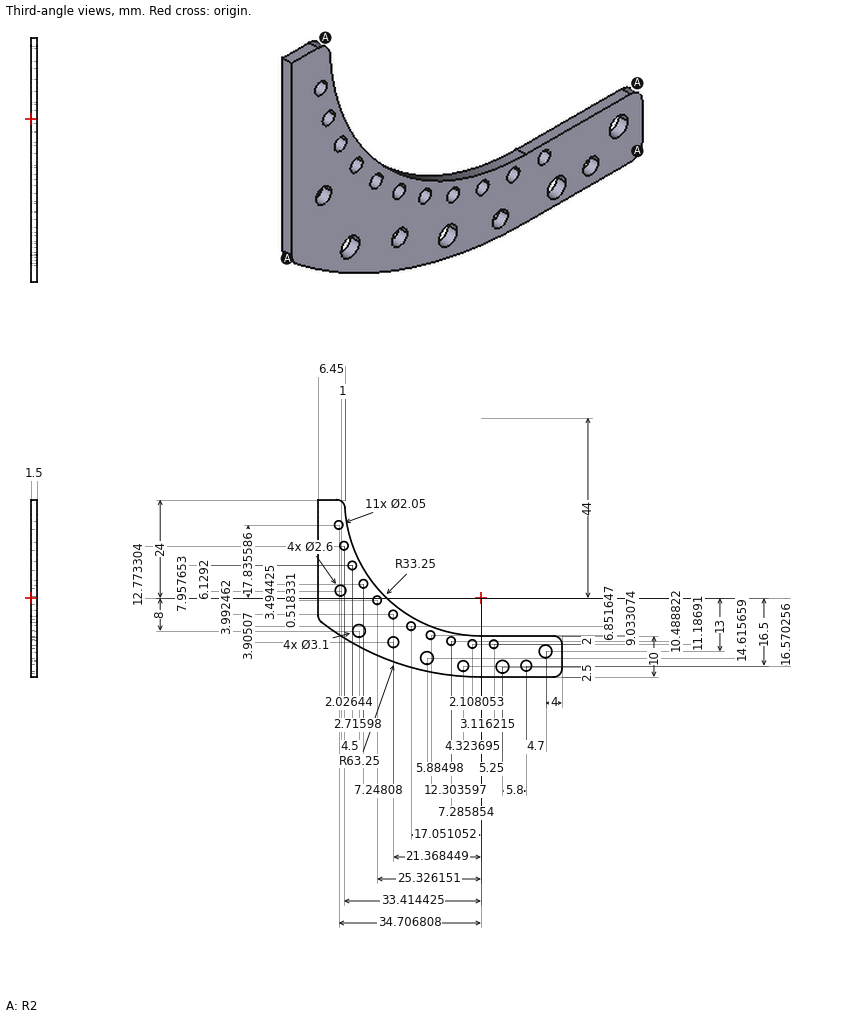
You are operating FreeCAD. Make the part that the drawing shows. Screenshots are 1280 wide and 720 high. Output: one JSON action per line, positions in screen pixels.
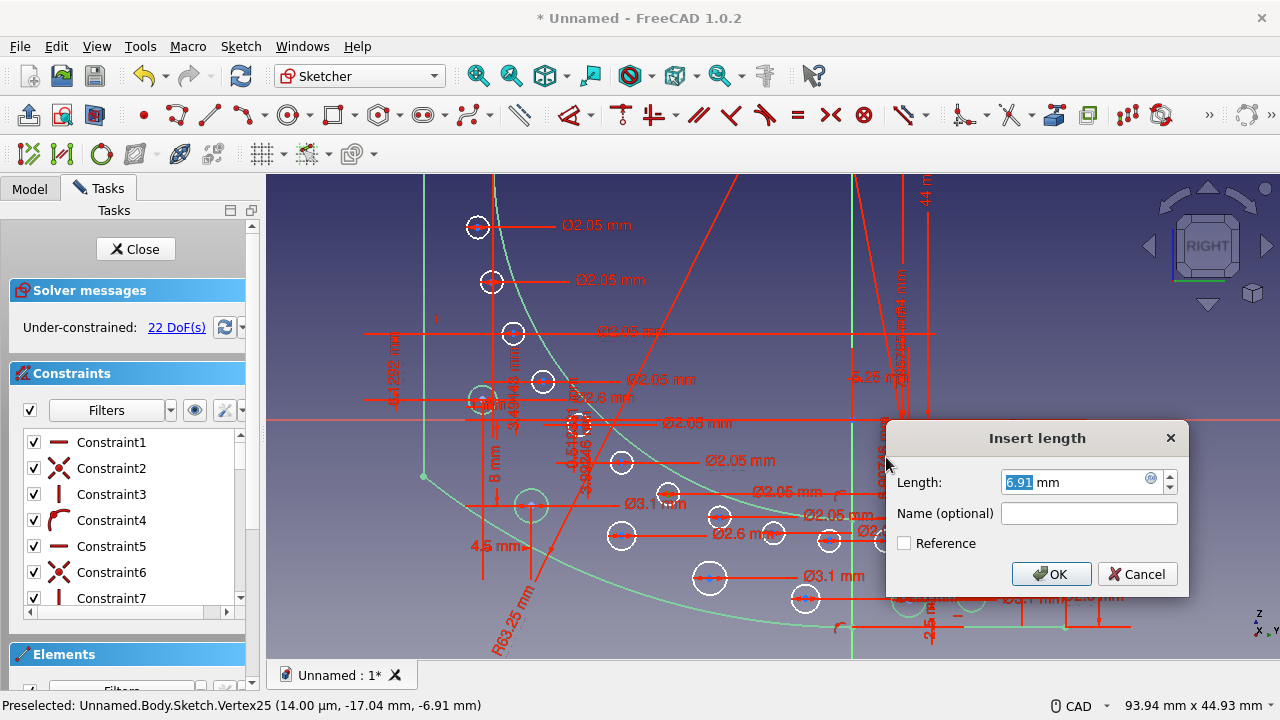
{"action": "type", "text": "6.851647"}
{"action": "key", "text": "Return"}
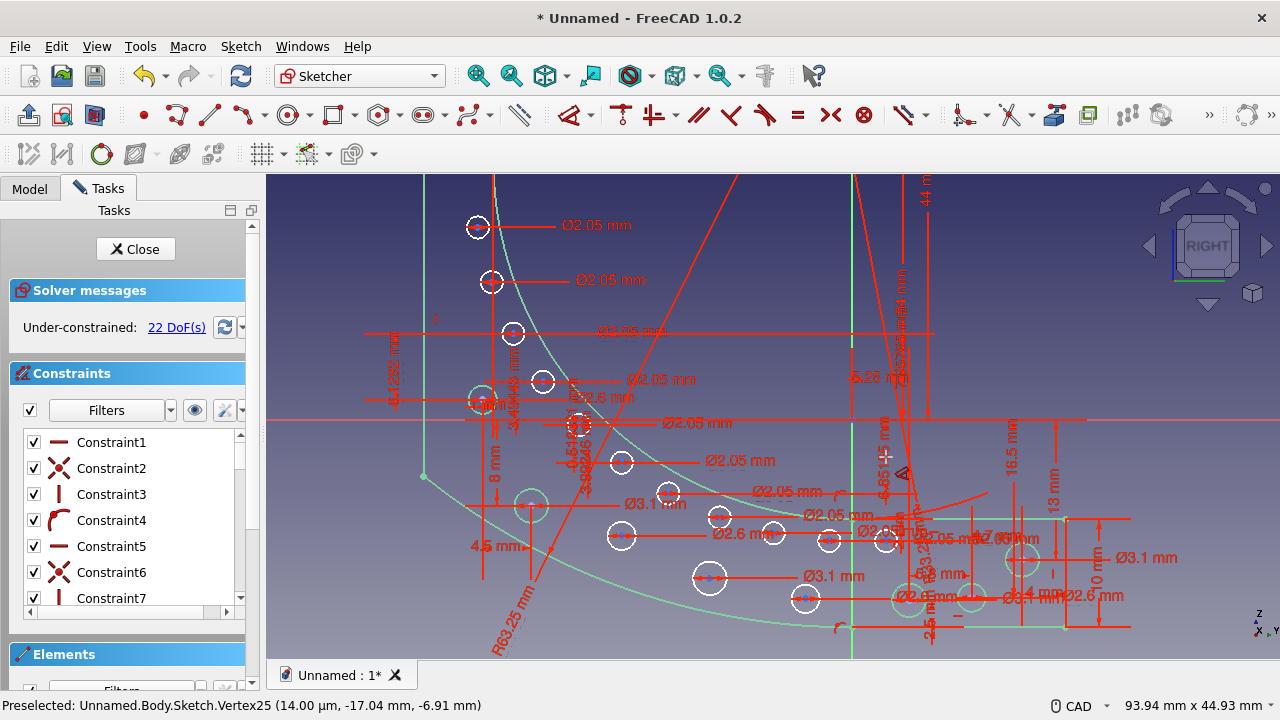
{"action": "left_click", "coordinate": [720, 517]}
{"action": "left_click", "coordinate": [886, 491]}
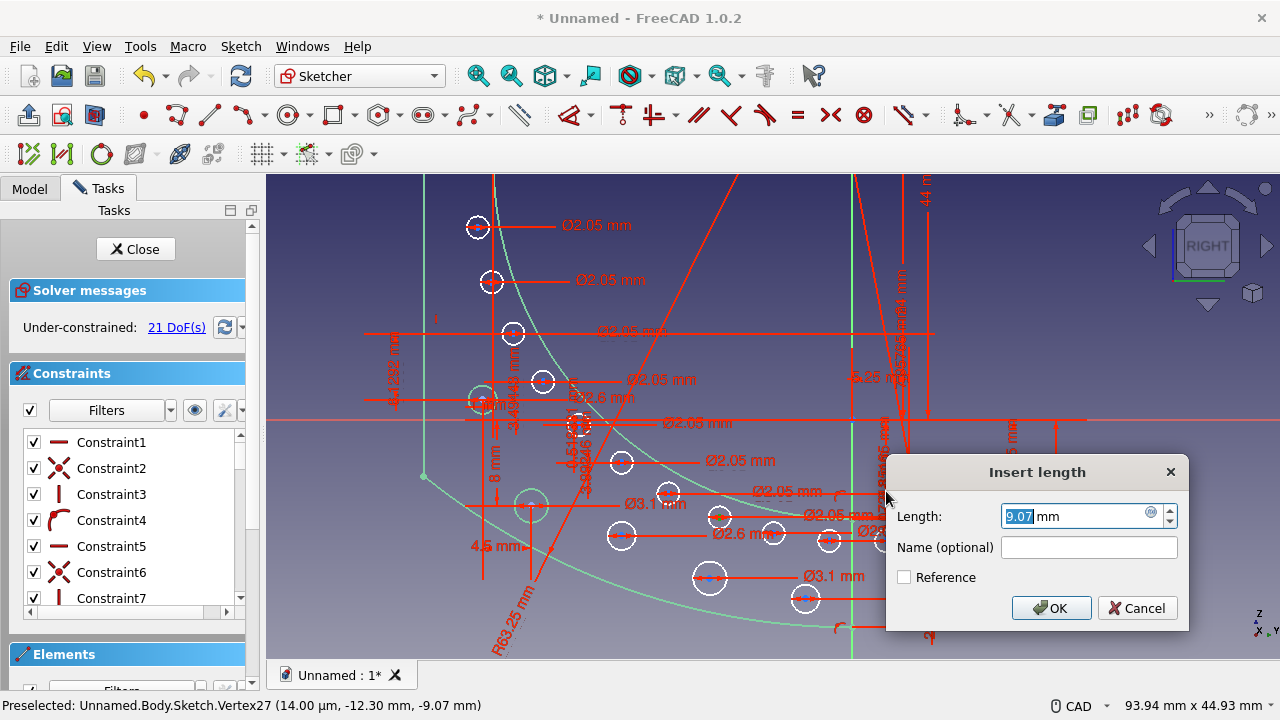
{"action": "type", "text": "9.033074"}
{"action": "key", "text": "Return"}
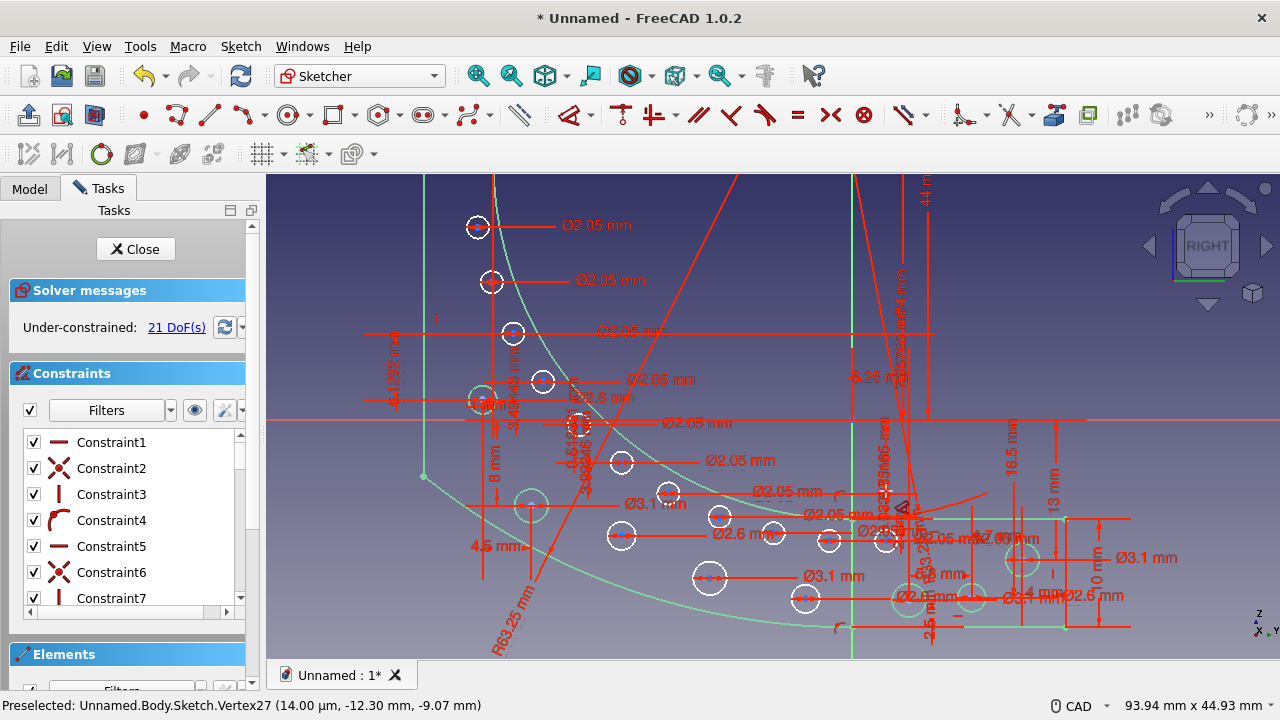
{"action": "left_click", "coordinate": [774, 533]}
{"action": "left_click", "coordinate": [813, 567]}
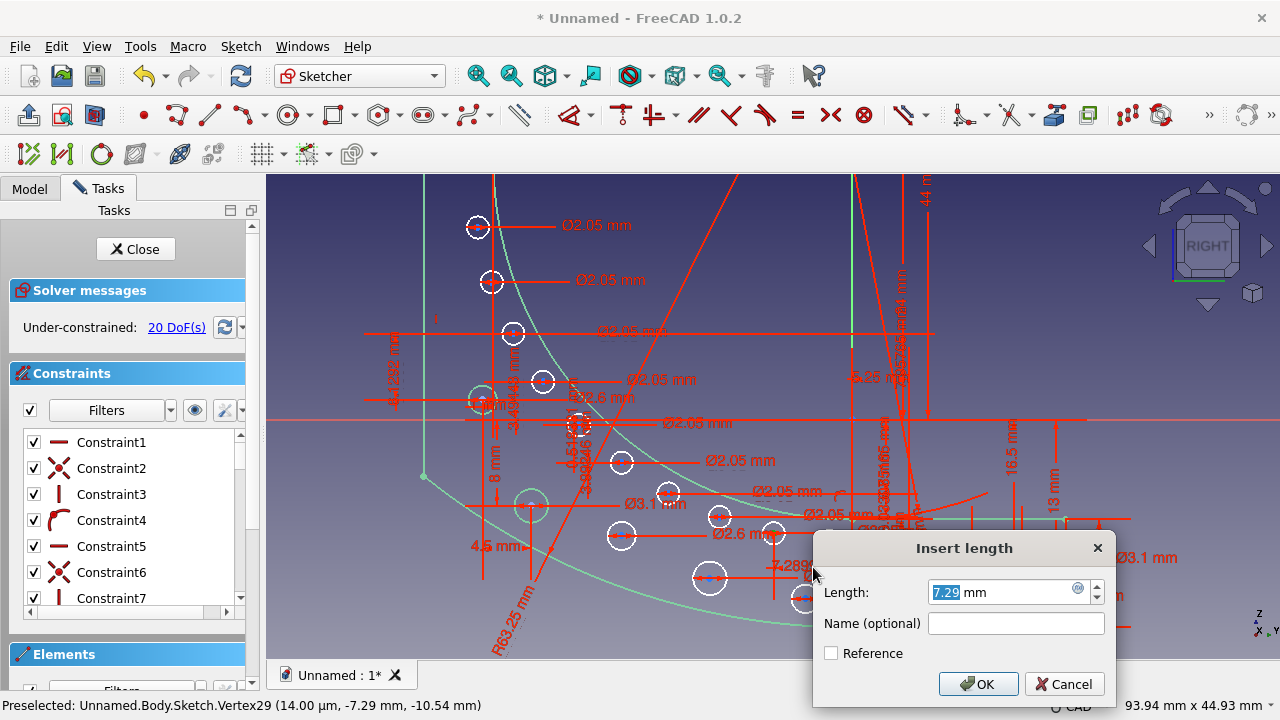
{"action": "type", "text": "7.285854"}
{"action": "key", "text": "Return"}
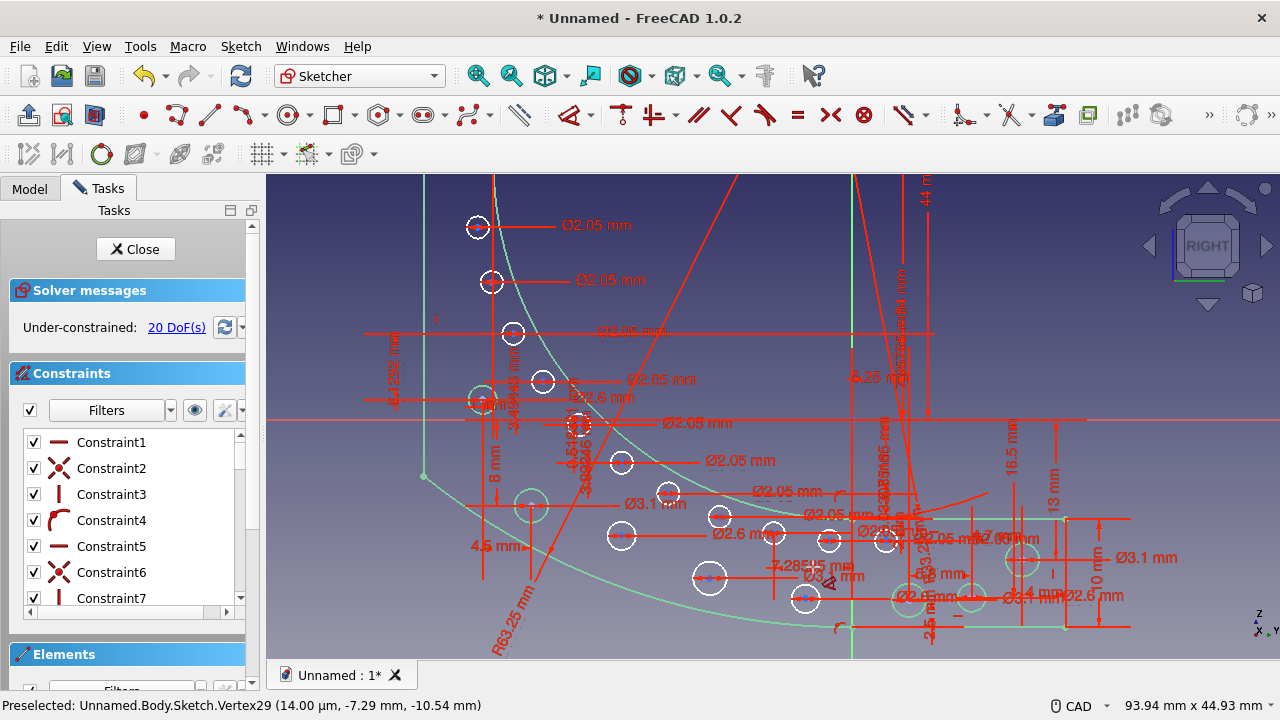
{"action": "left_click", "coordinate": [806, 599]}
{"action": "left_click", "coordinate": [829, 338]}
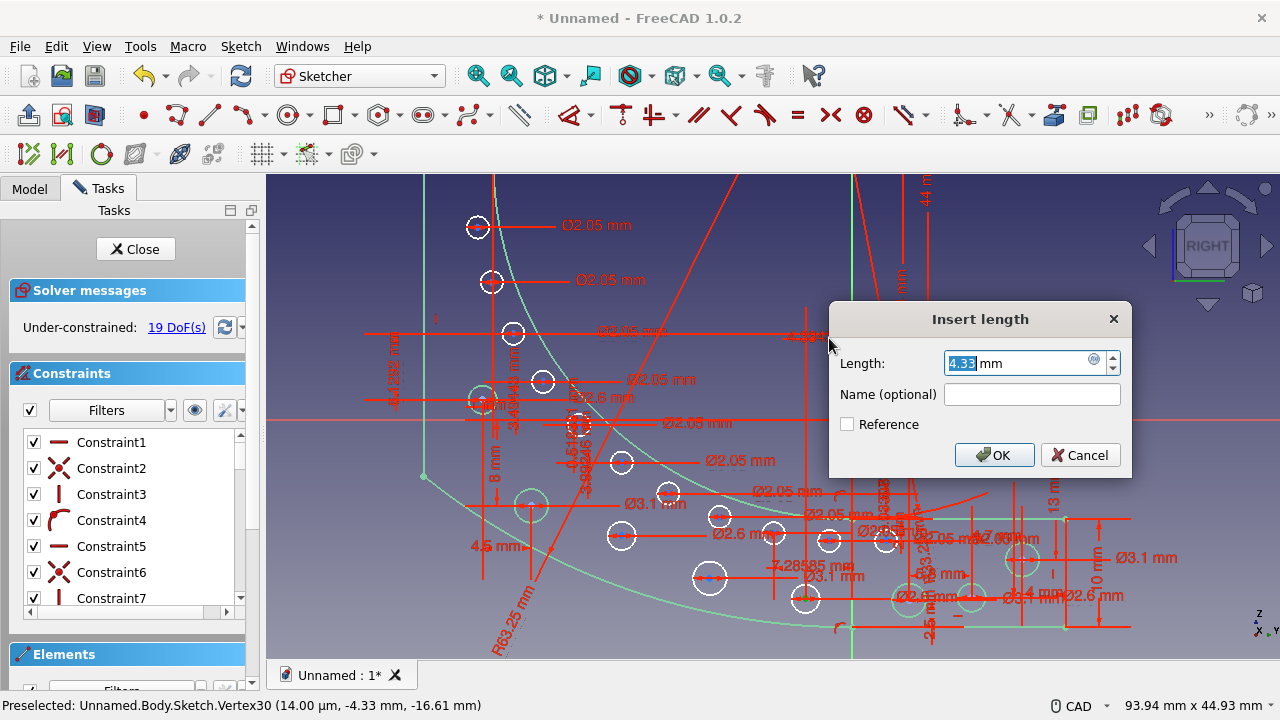
{"action": "type", "text": "4.323695"}
{"action": "key", "text": "Return"}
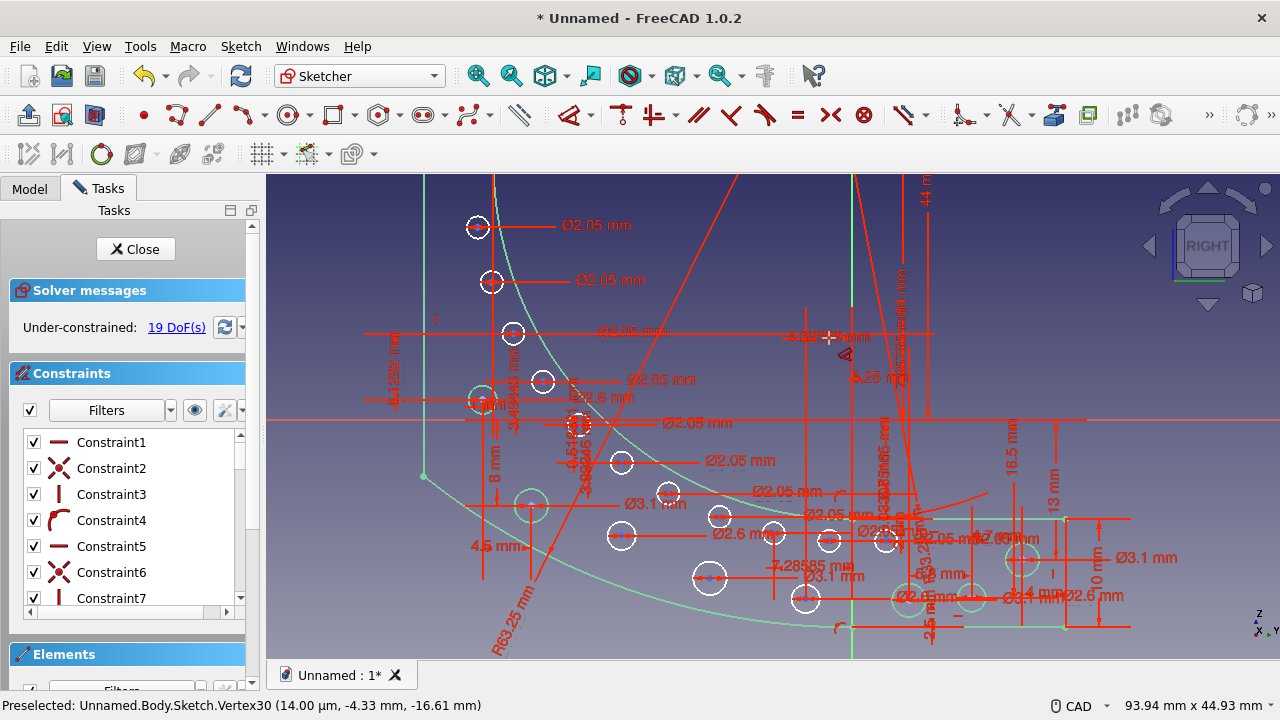
{"action": "scroll", "coordinate": [829, 541], "scroll_direction": "up", "scroll_amount": 3}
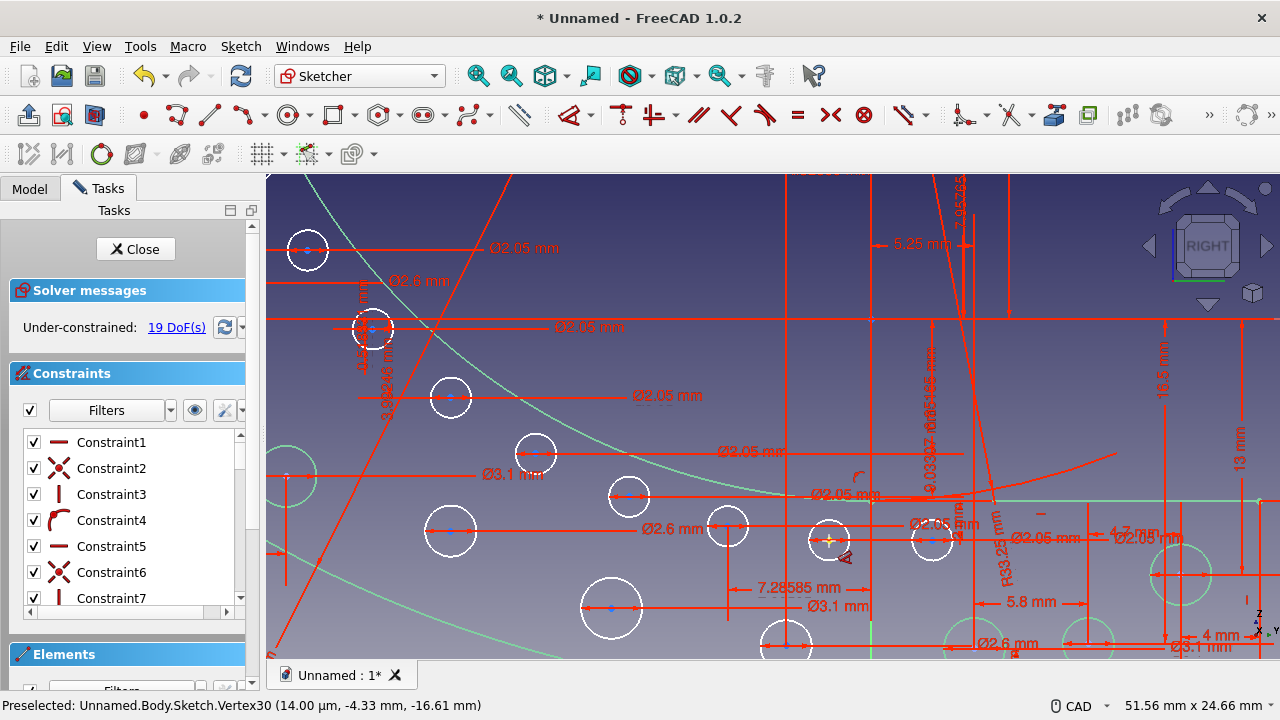
{"action": "left_click", "coordinate": [829, 540]}
{"action": "left_click", "coordinate": [850, 285]}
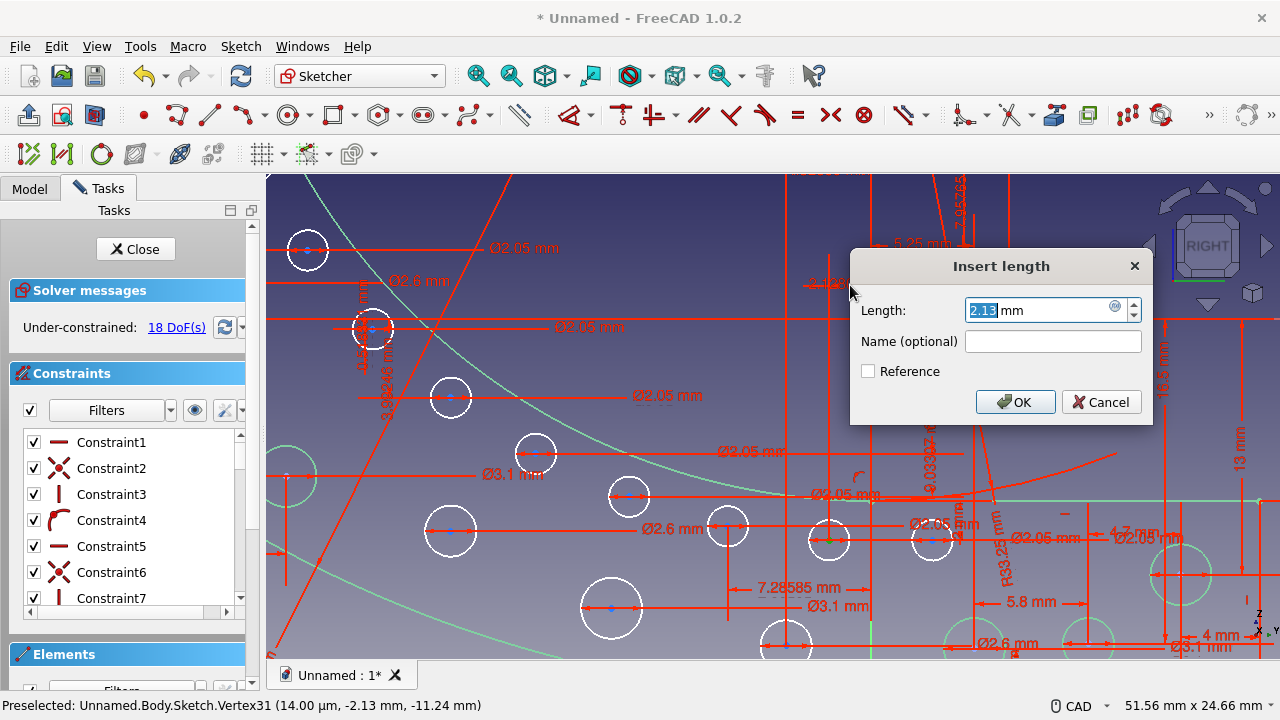
{"action": "type", "text": "2.108053"}
{"action": "key", "text": "Return"}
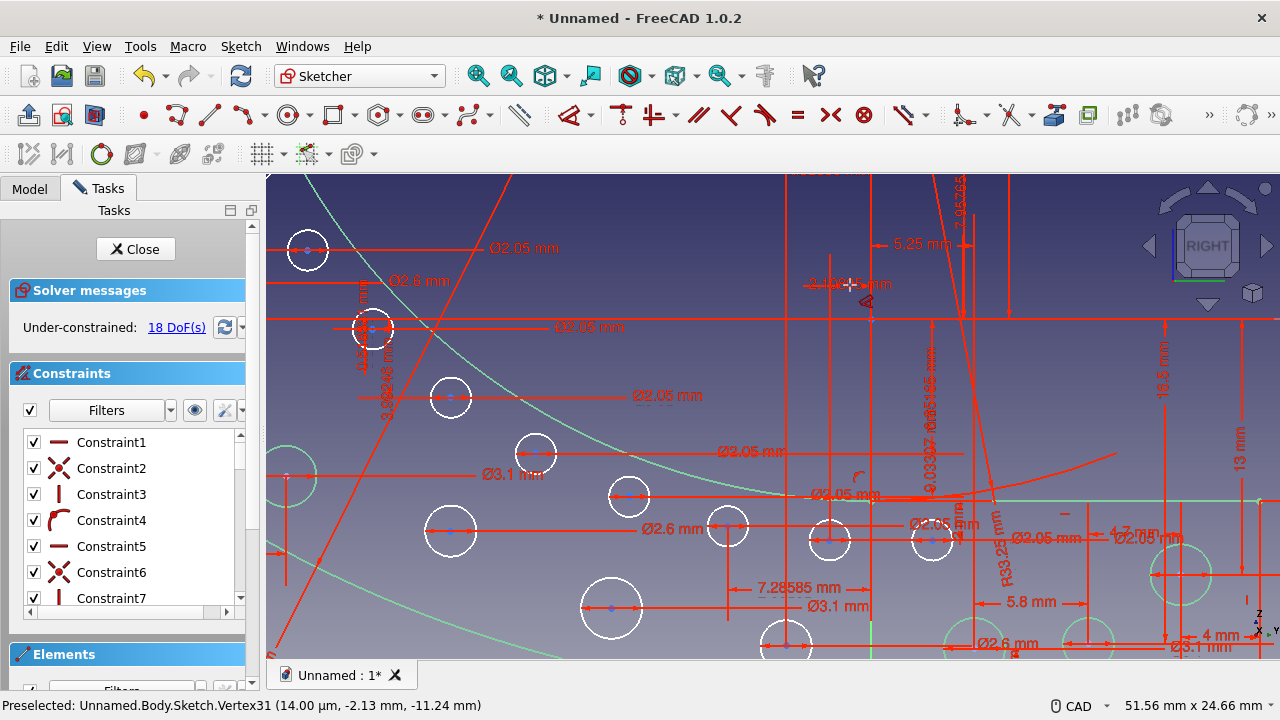
{"action": "left_click", "coordinate": [830, 540]}
{"action": "left_click", "coordinate": [905, 481]}